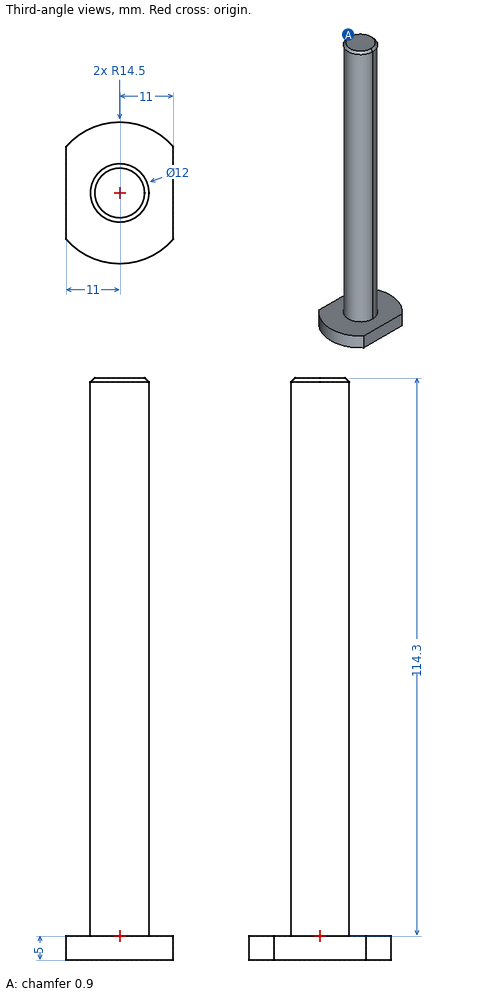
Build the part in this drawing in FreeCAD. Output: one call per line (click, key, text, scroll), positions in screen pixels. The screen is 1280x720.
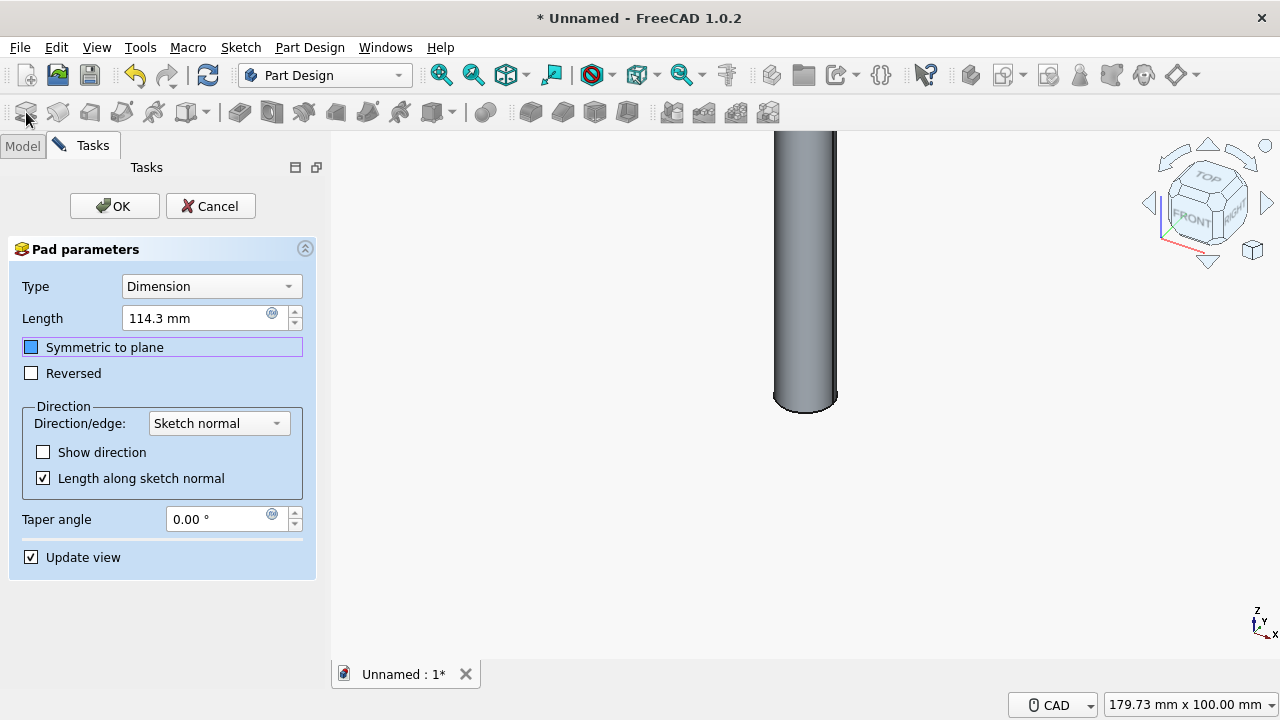
click(115, 206)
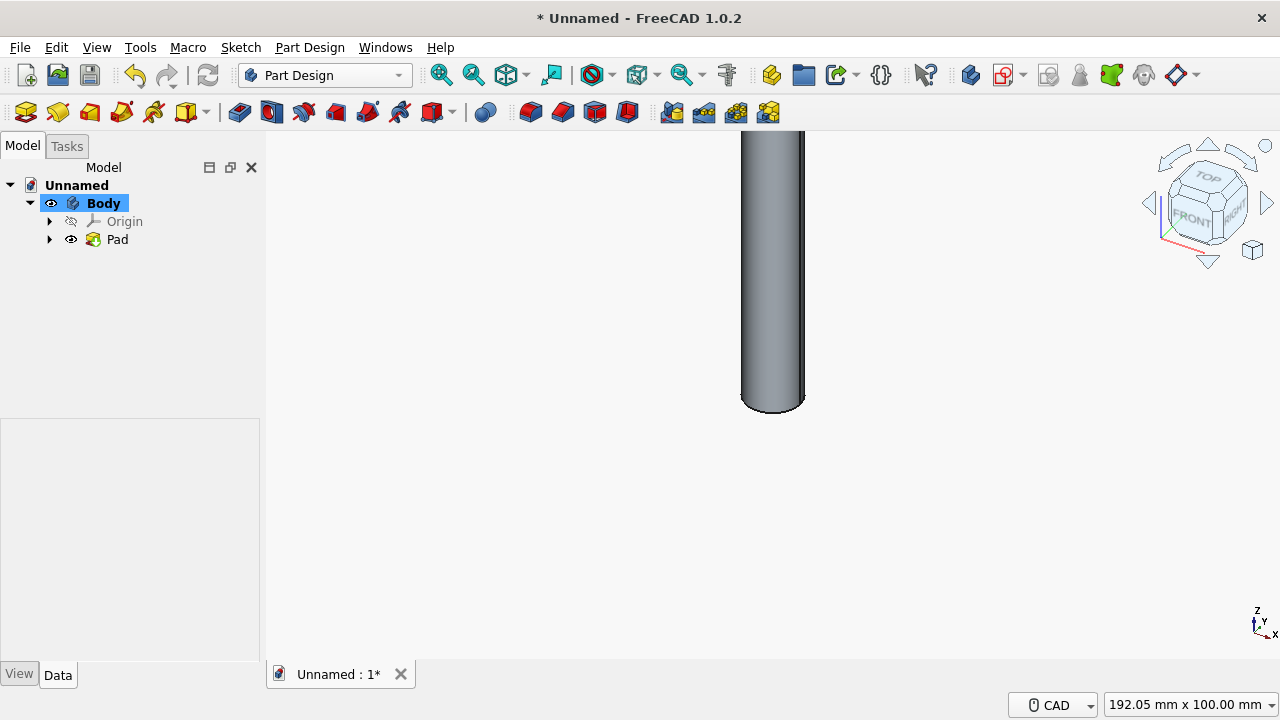
click(442, 76)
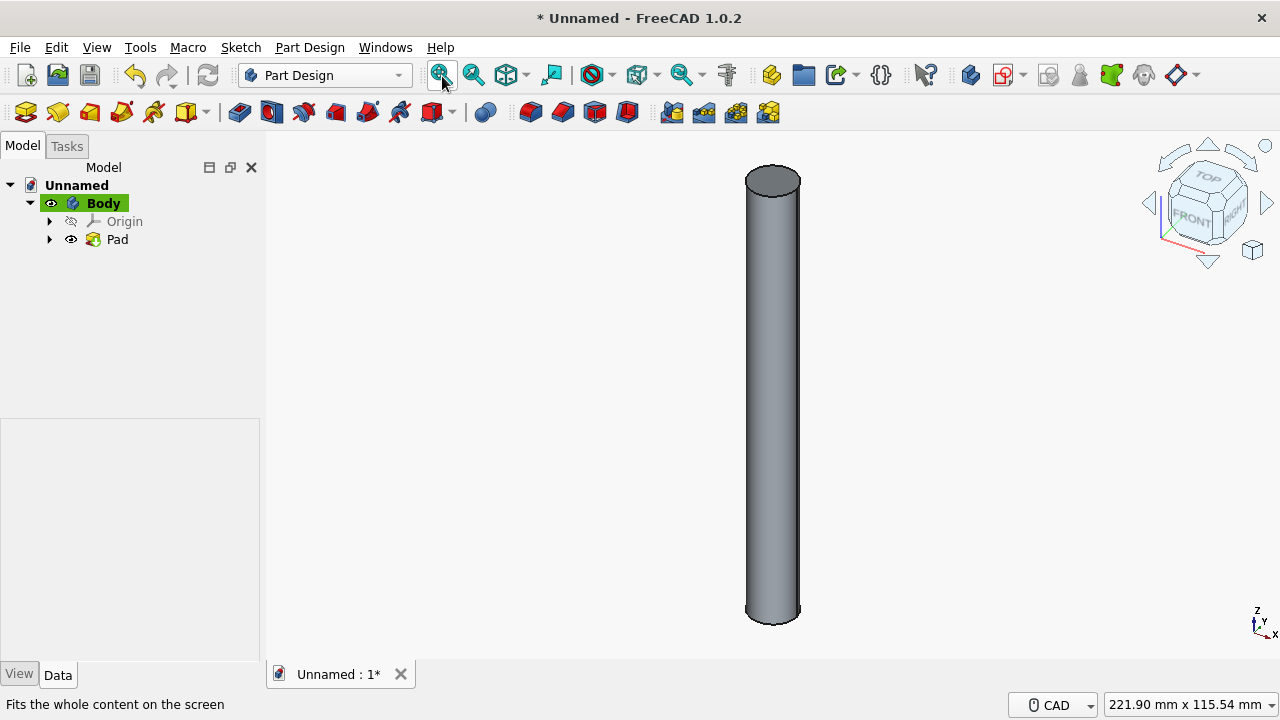
click(746, 182)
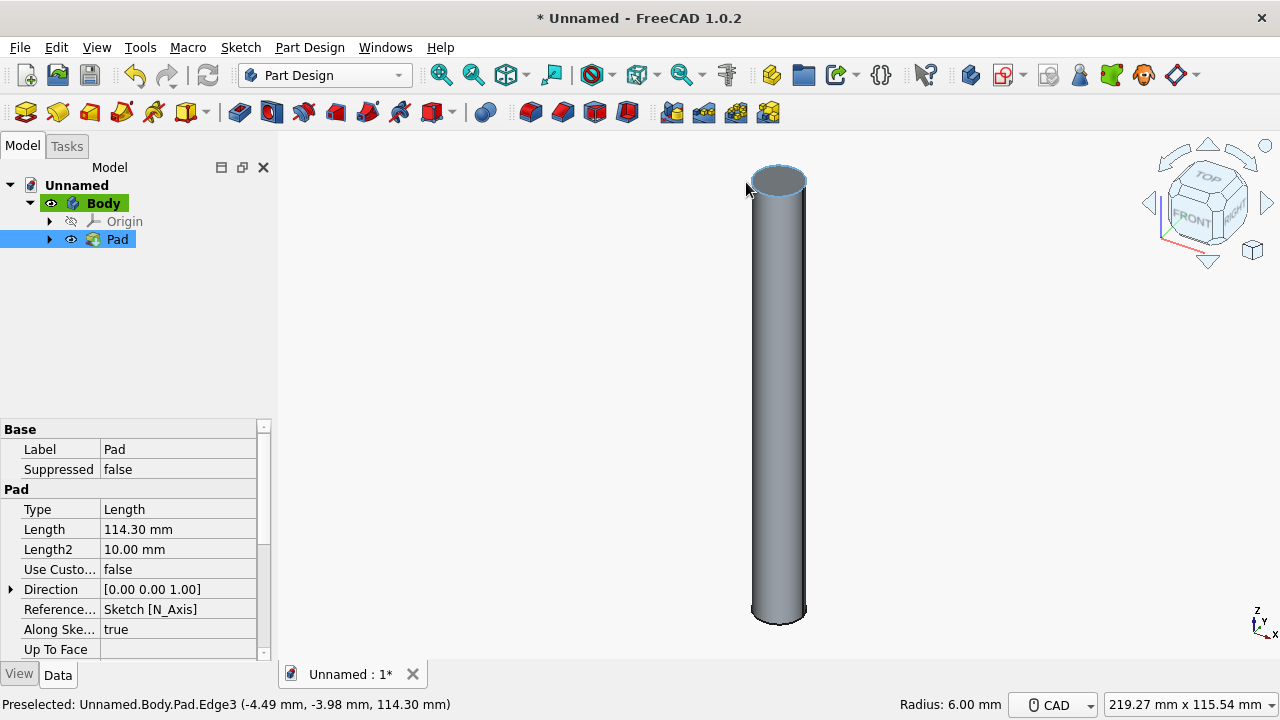
click(564, 112)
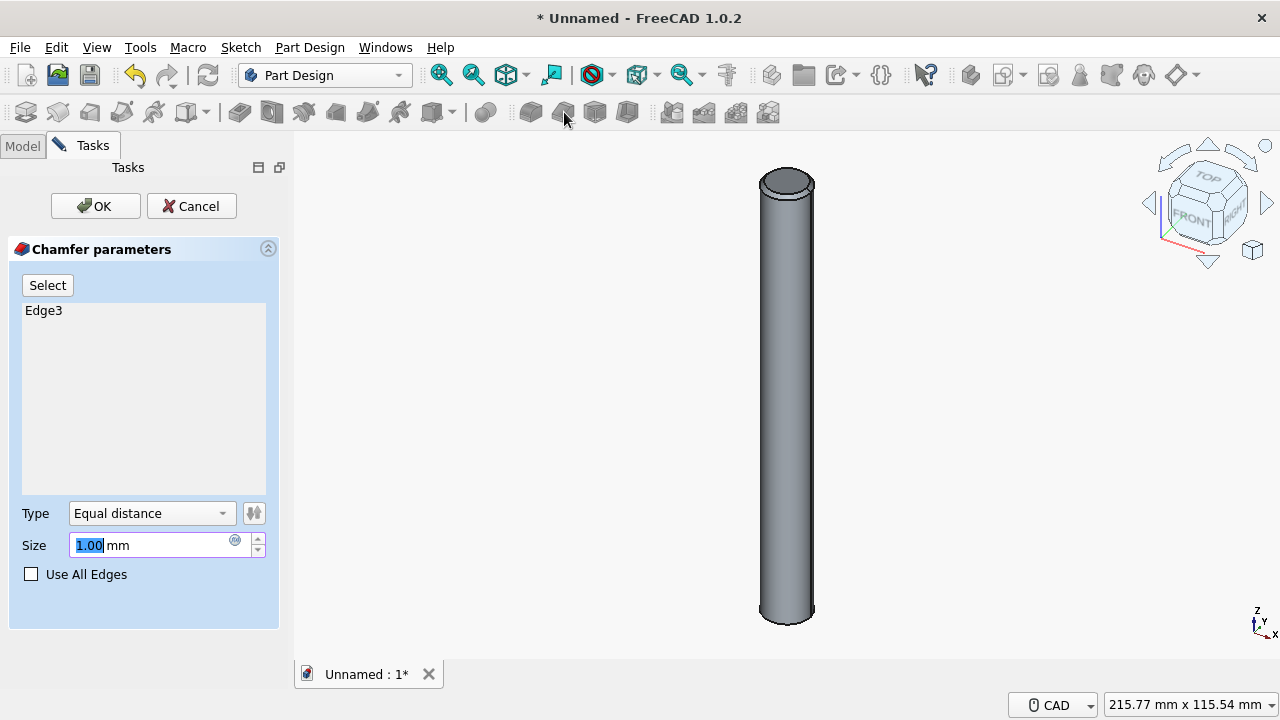
text(0.9)
key(Tab)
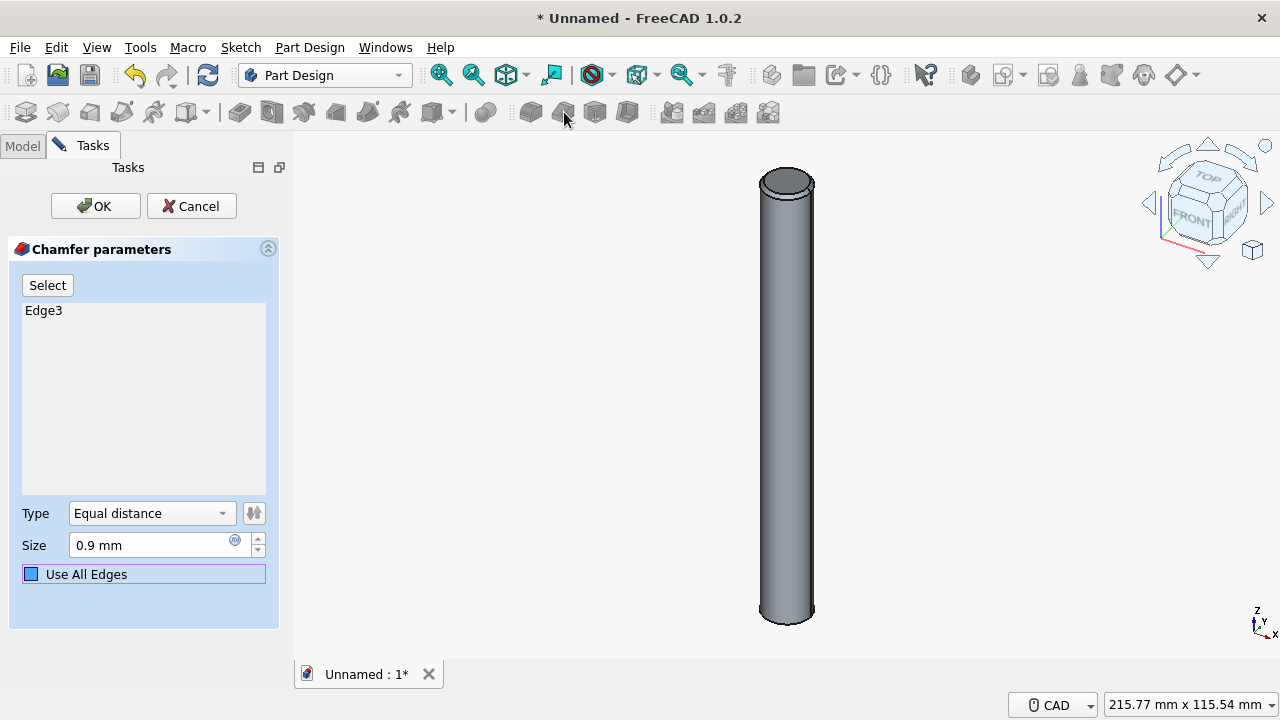
click(96, 206)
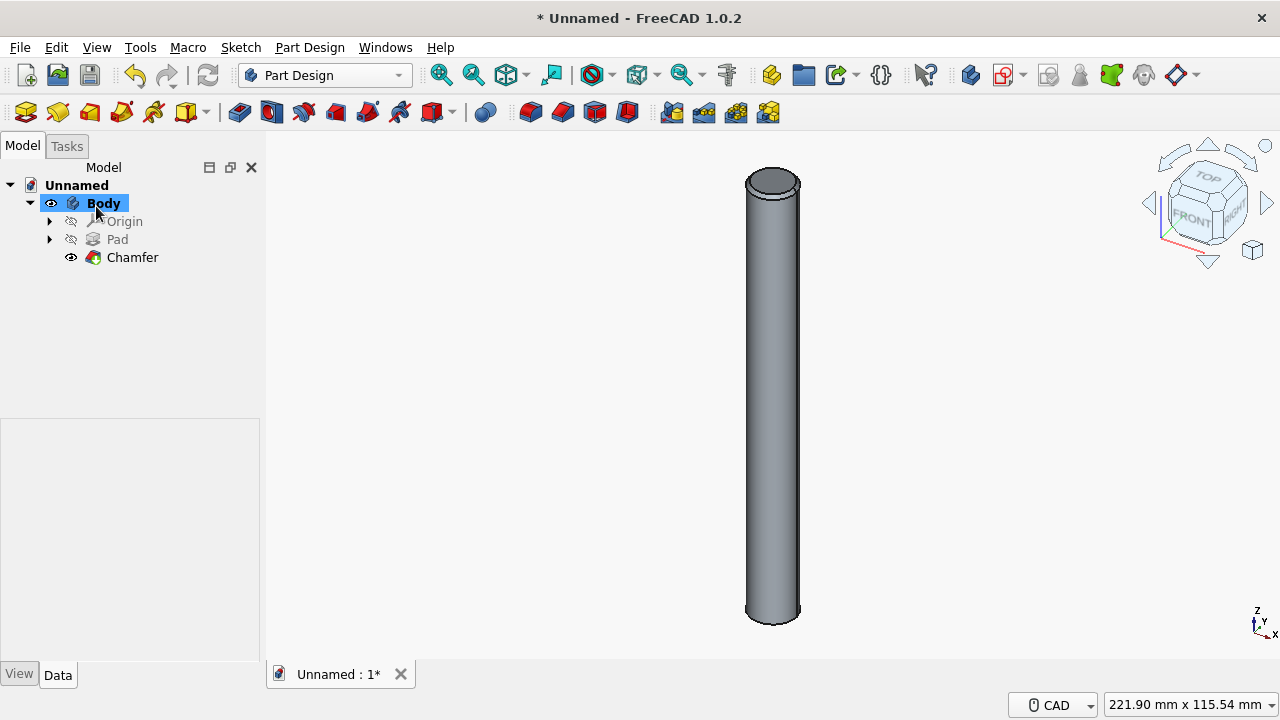
click(1004, 76)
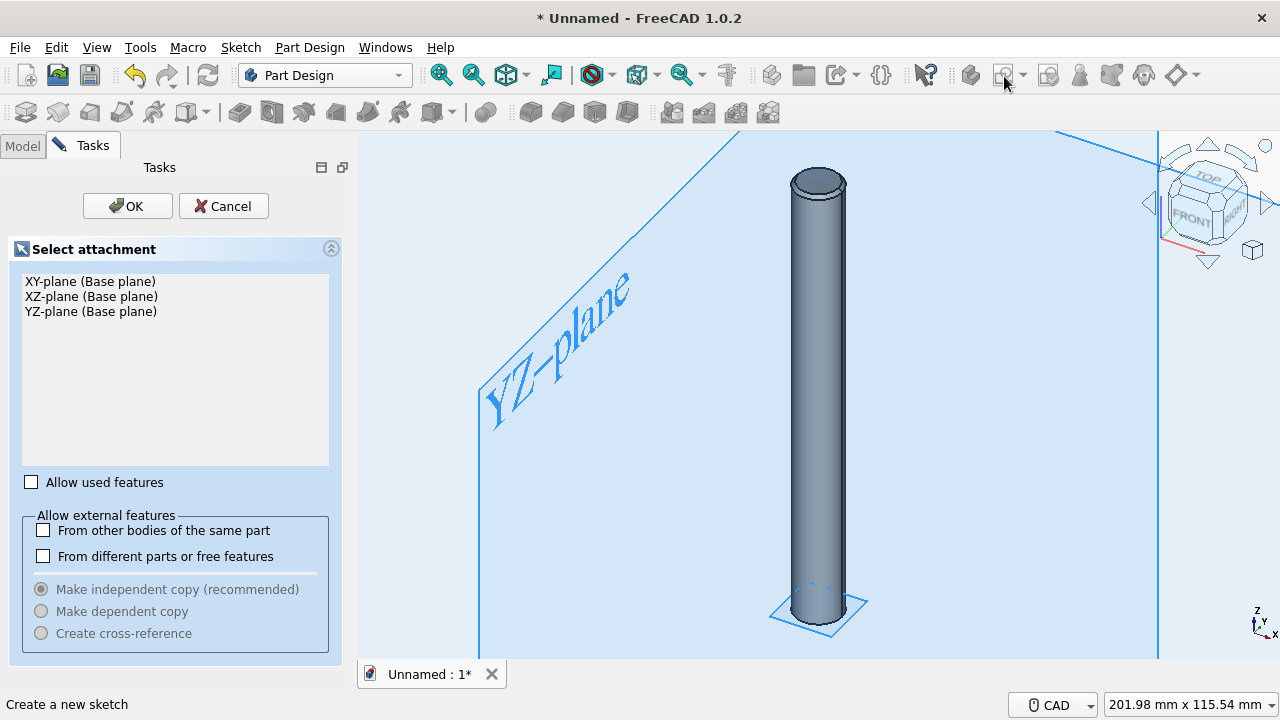
click(82, 282)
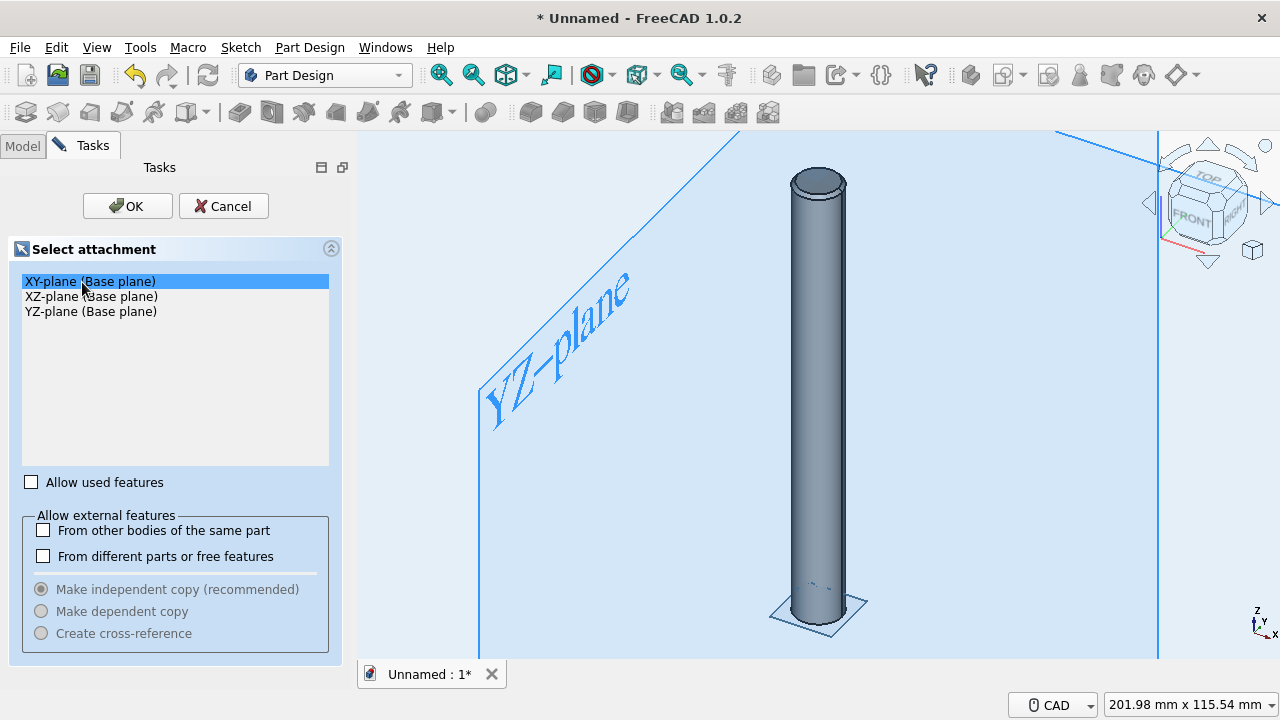
click(128, 206)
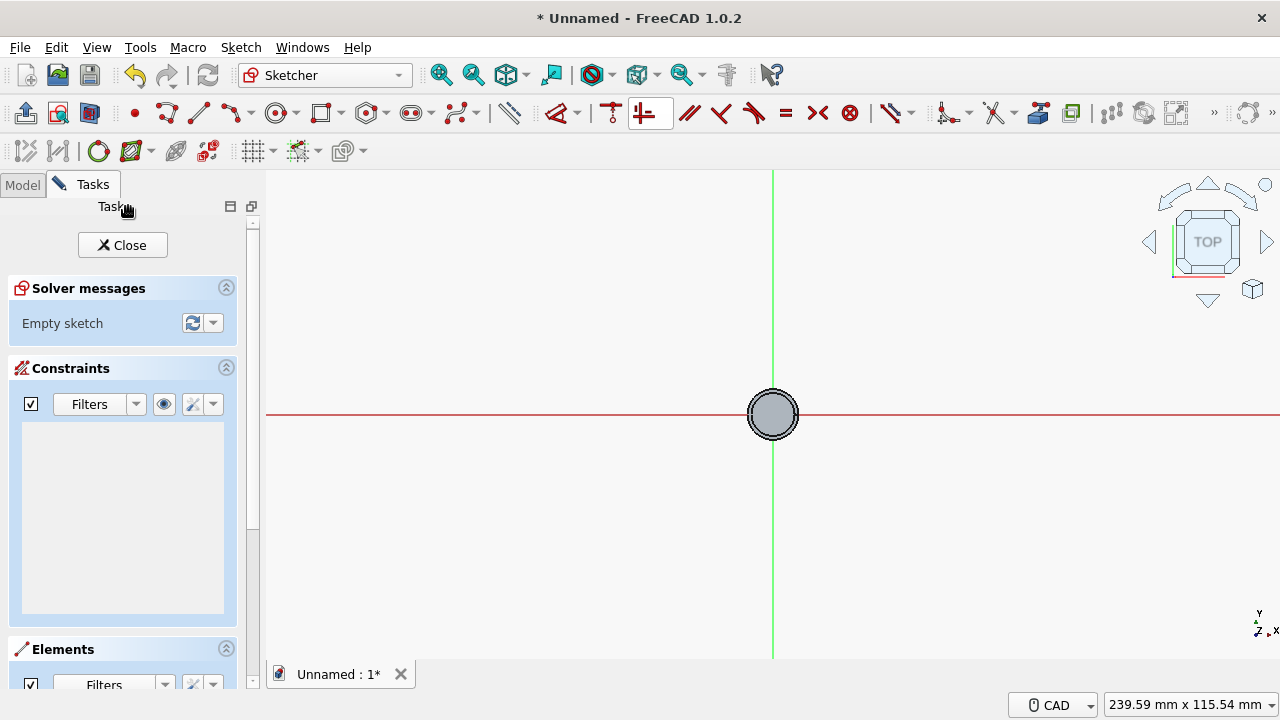
click(90, 114)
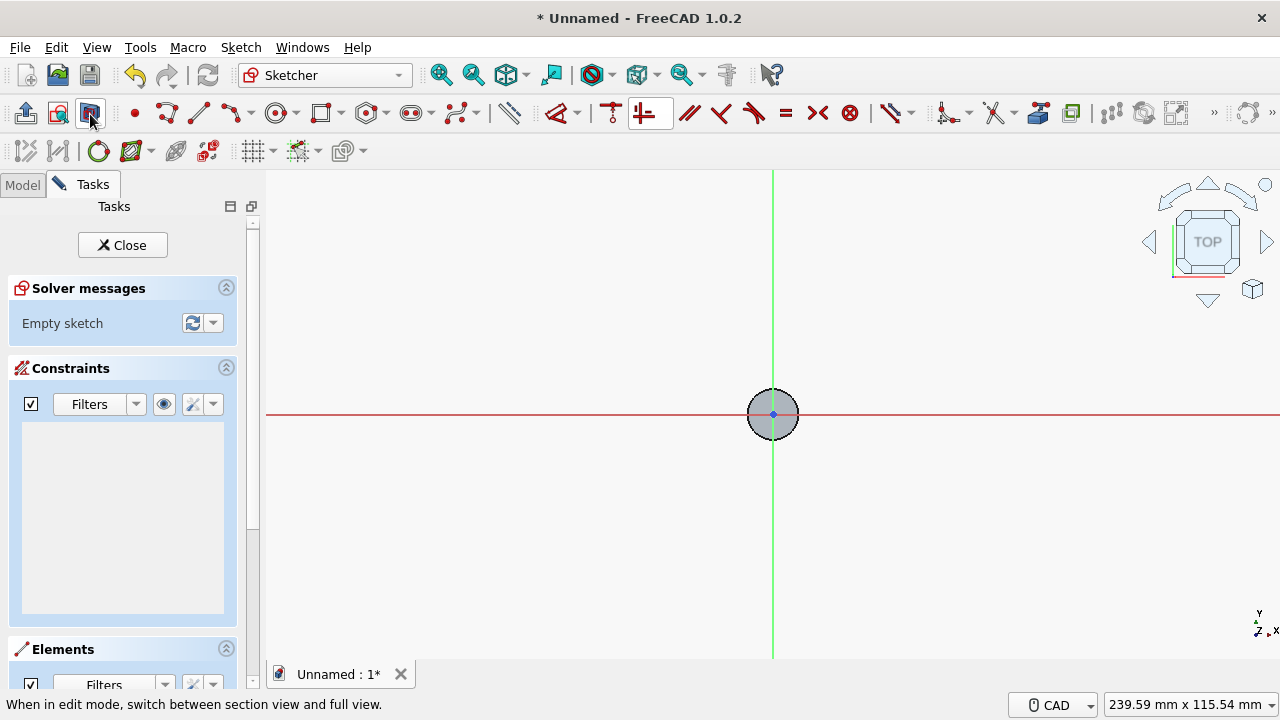
scroll(813, 415, up, 5)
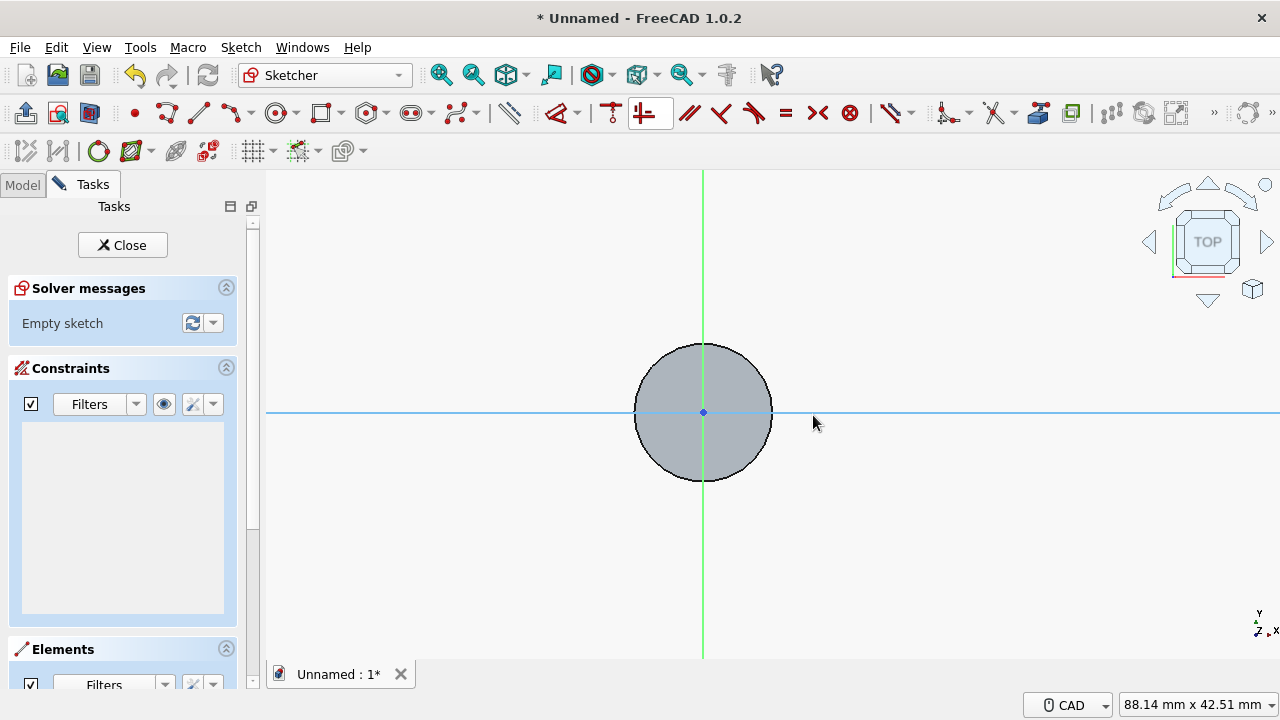
click(200, 114)